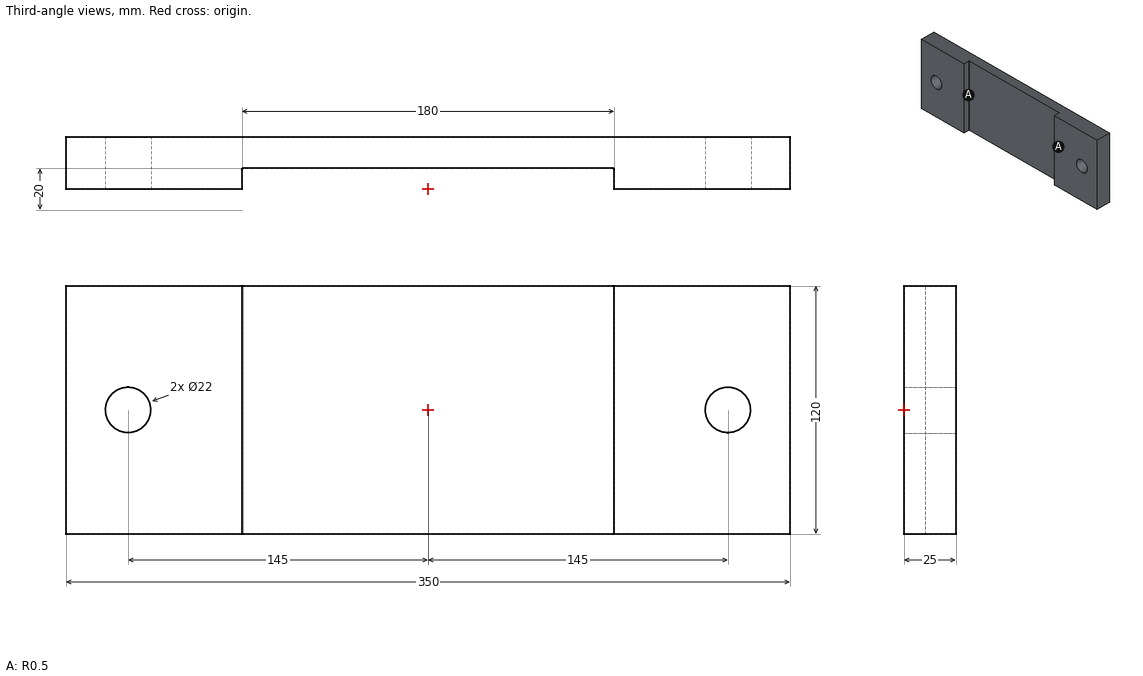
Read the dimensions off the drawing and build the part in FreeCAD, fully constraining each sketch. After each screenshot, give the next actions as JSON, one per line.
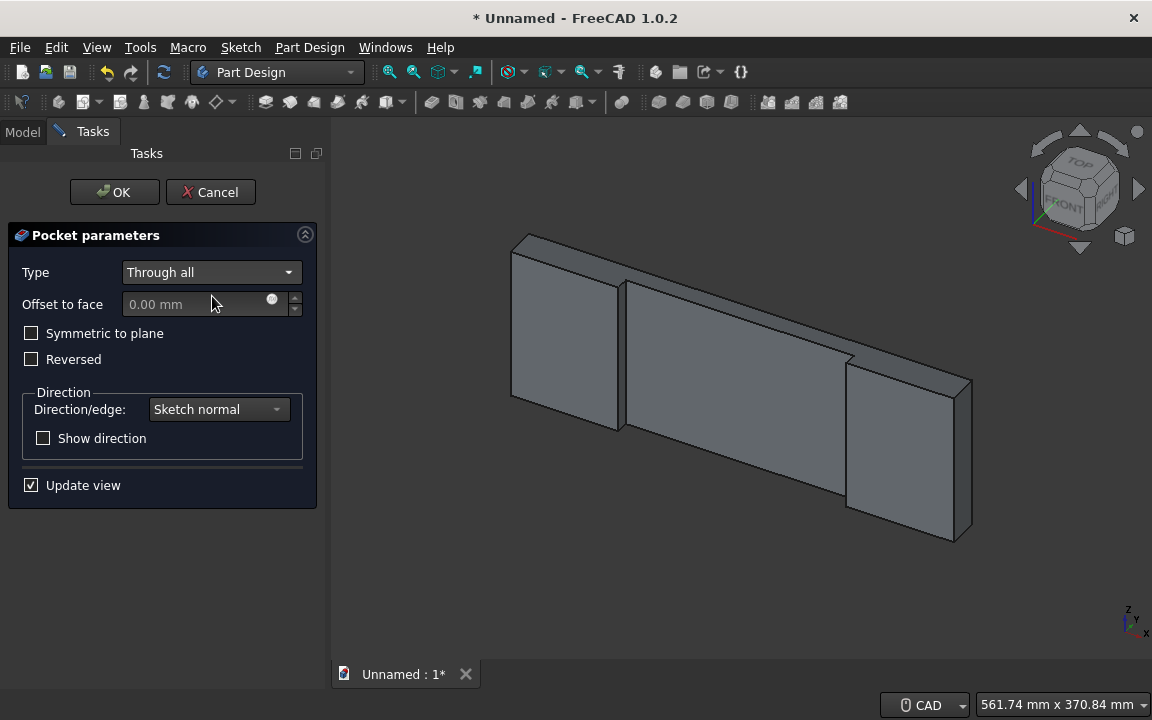
{"action": "left_click", "coordinate": [115, 192]}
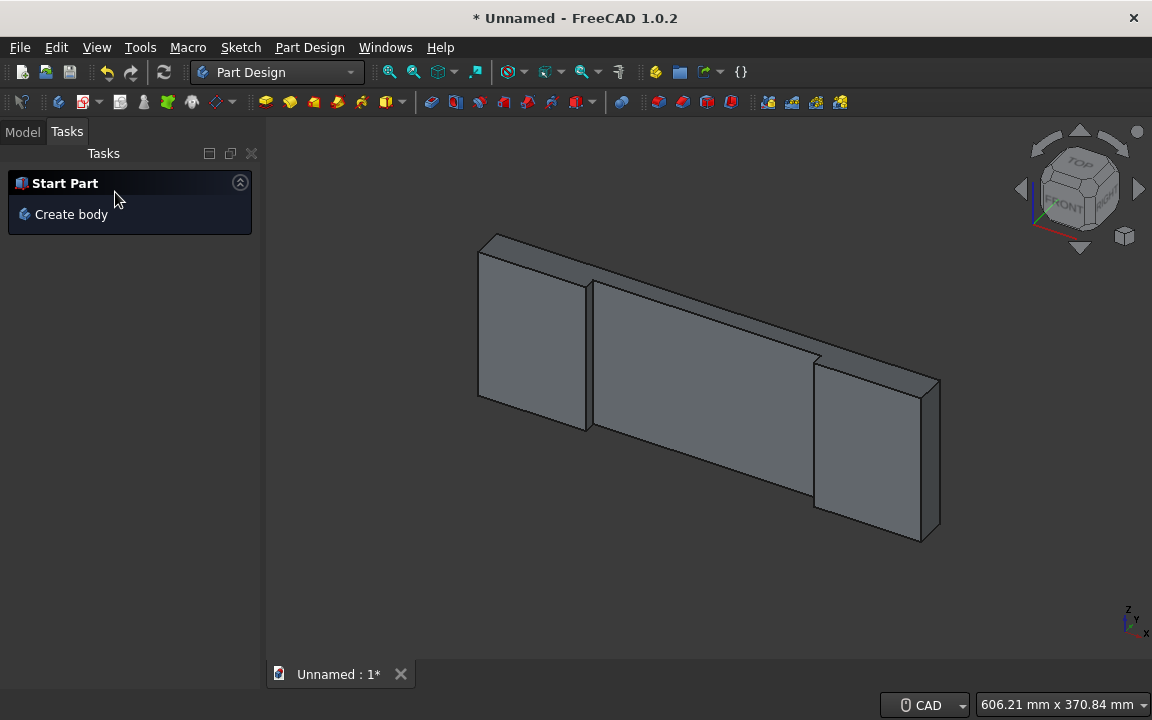
{"action": "key", "text": "4"}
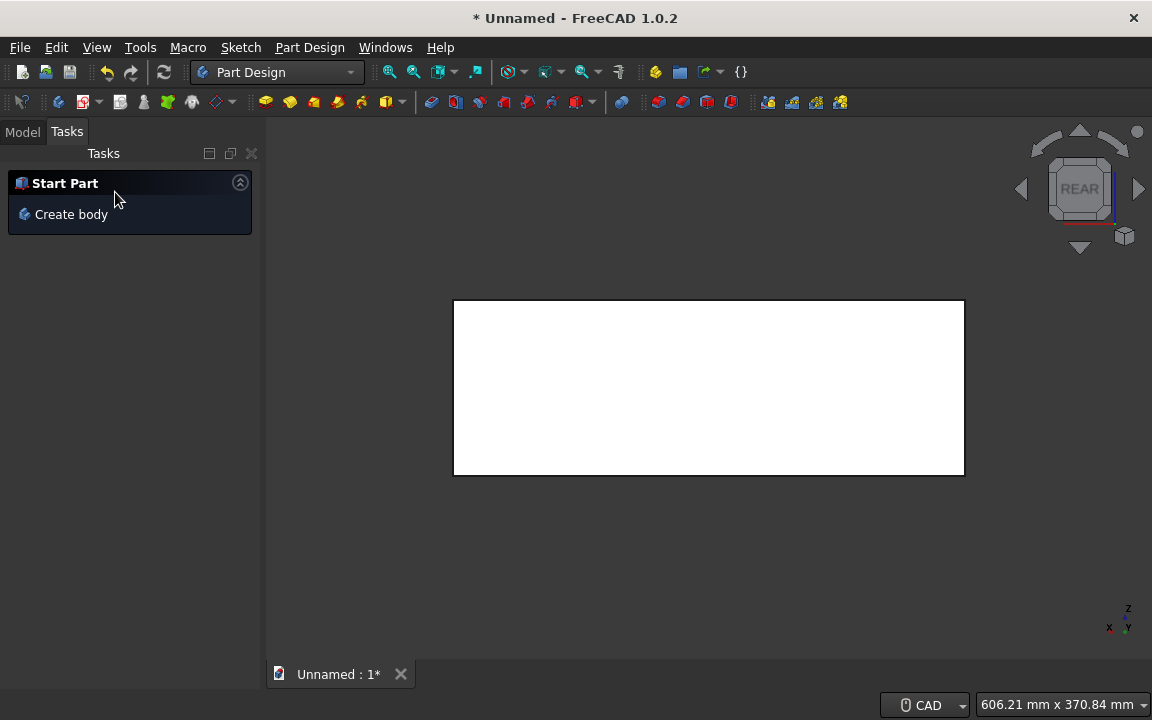
{"action": "left_click", "coordinate": [563, 387]}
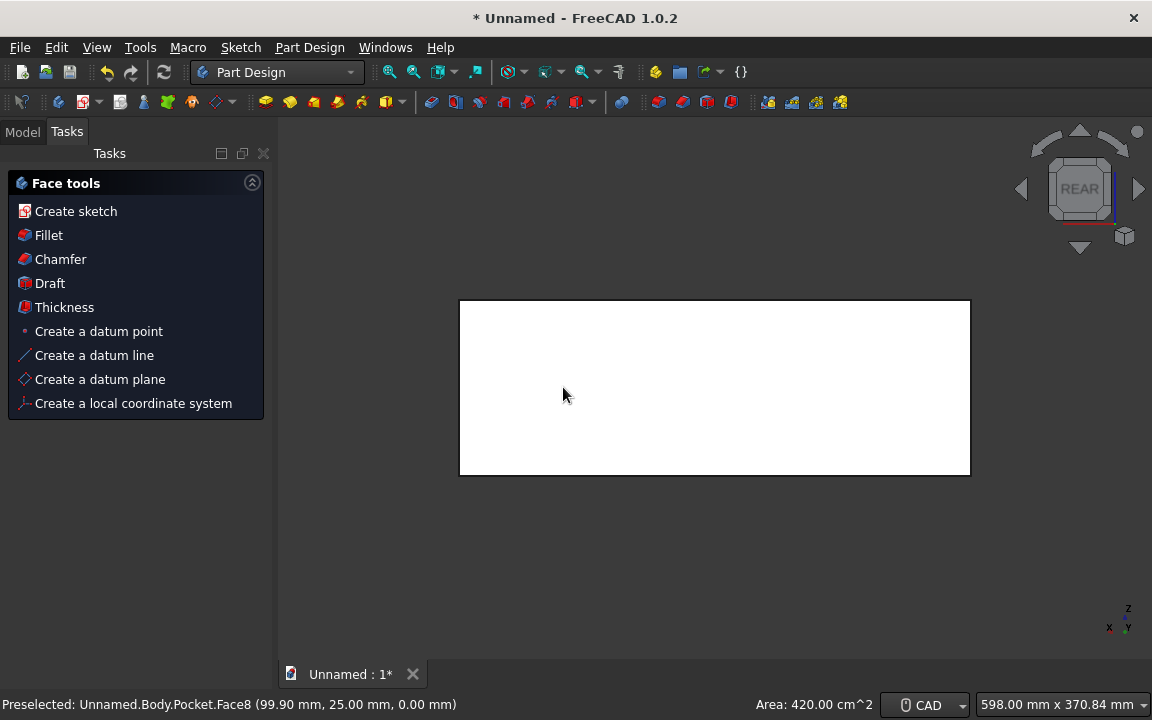
{"action": "left_click", "coordinate": [84, 102]}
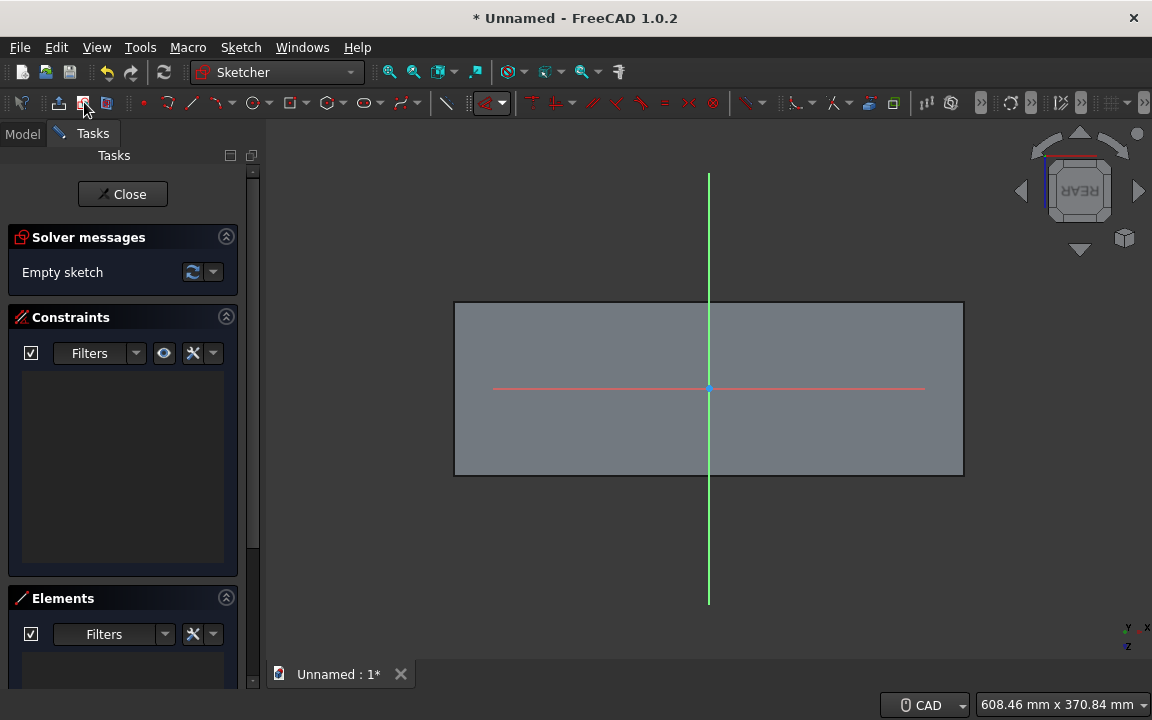
{"action": "left_click", "coordinate": [254, 104]}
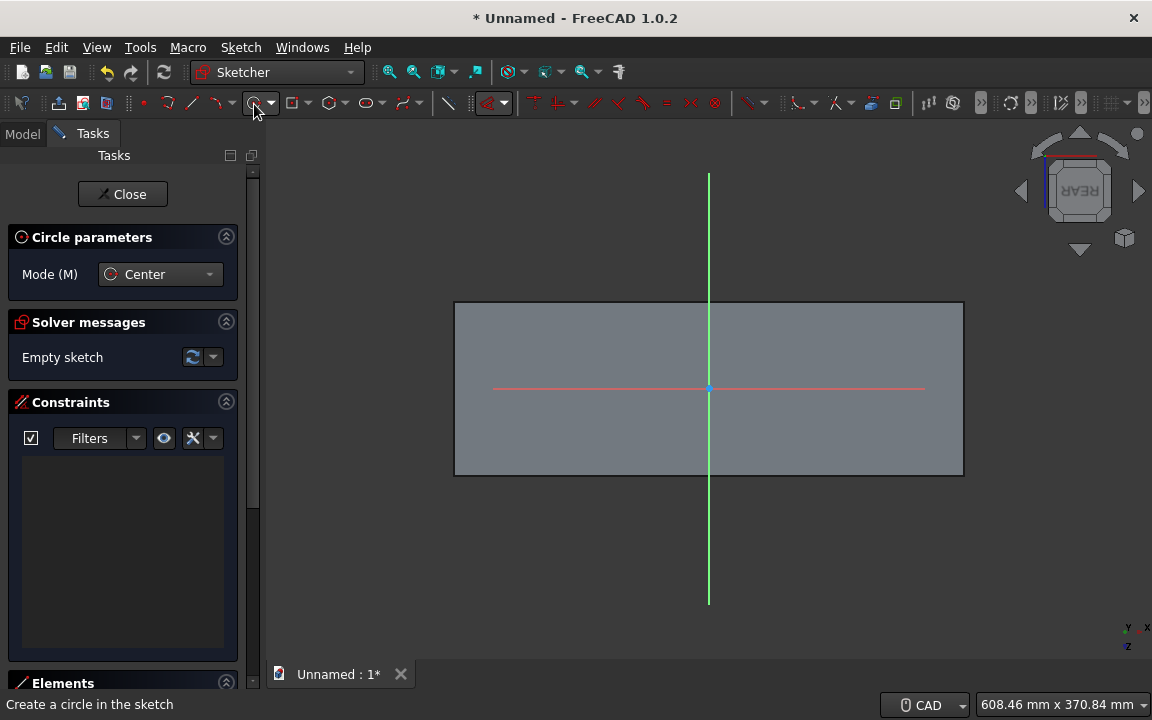
{"action": "scroll", "coordinate": [498, 389], "scroll_direction": "up", "scroll_amount": 2}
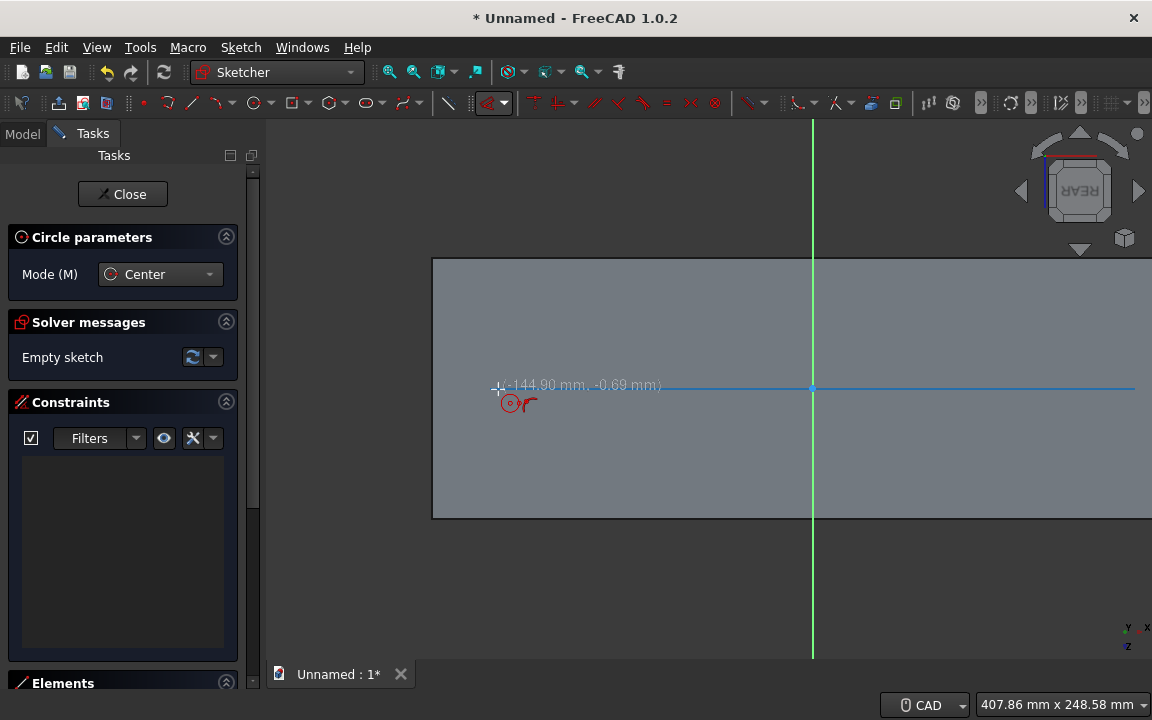
{"action": "left_click", "coordinate": [498, 389]}
{"action": "mouse_move", "coordinate": [515, 372]}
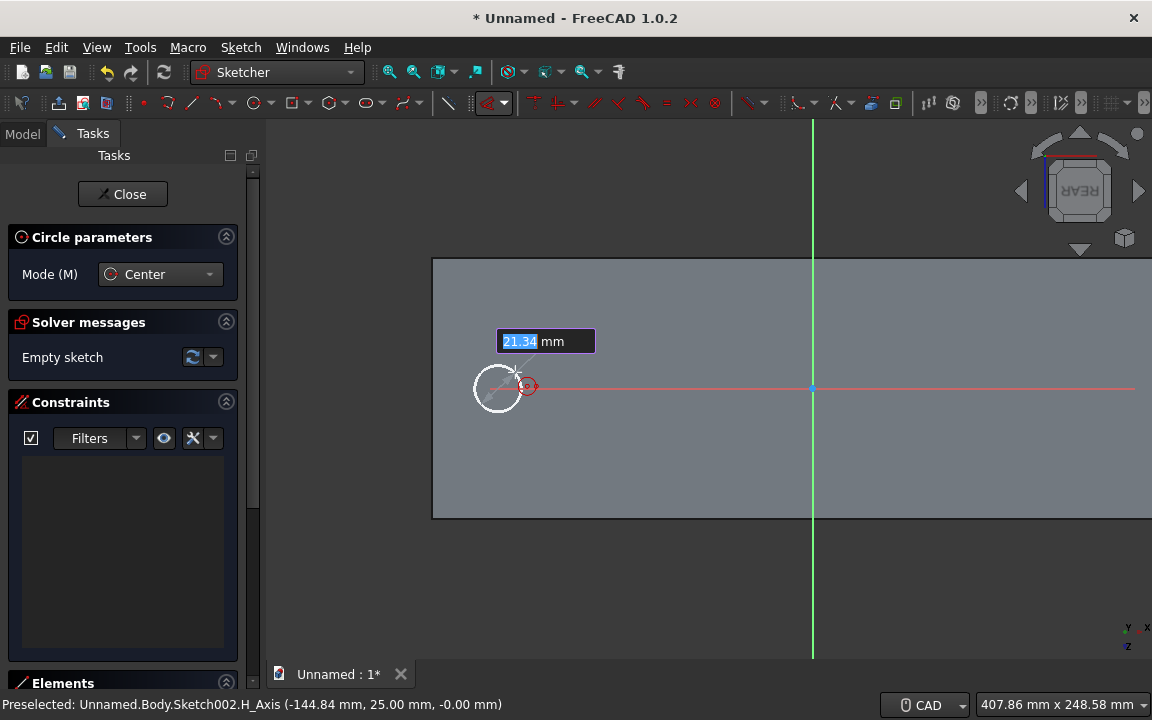
{"action": "type", "text": "22"}
{"action": "key", "text": "Return"}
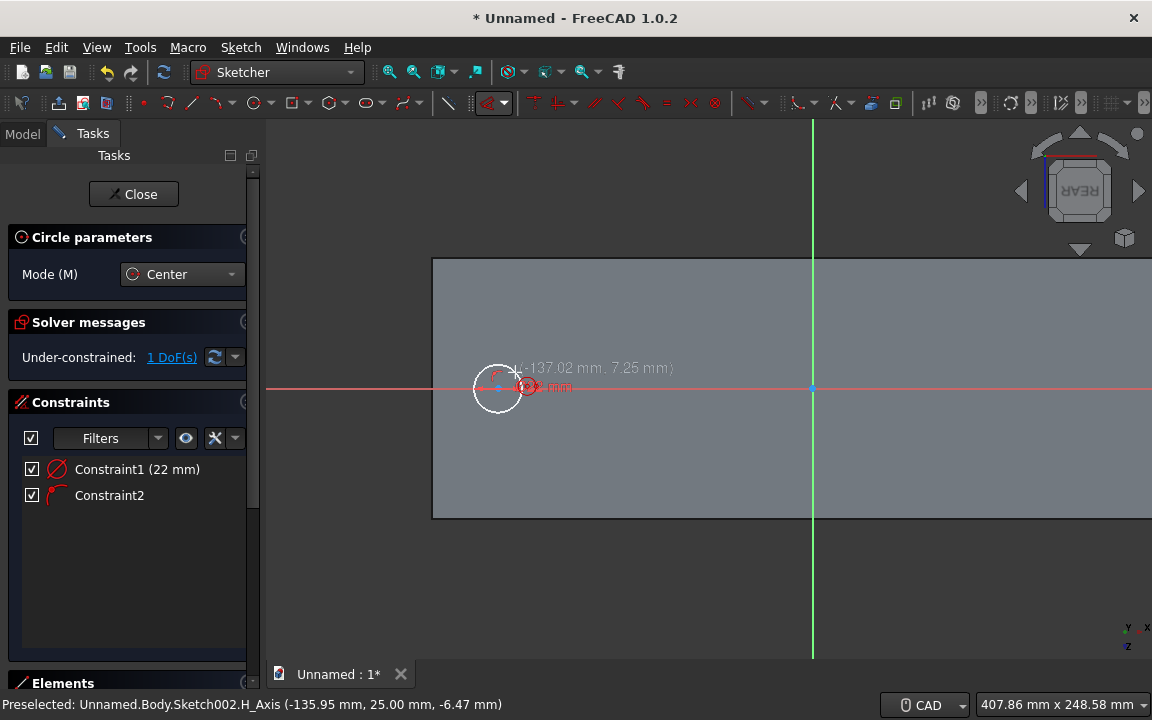
{"action": "scroll", "coordinate": [294, 390], "scroll_direction": "down", "scroll_amount": 2}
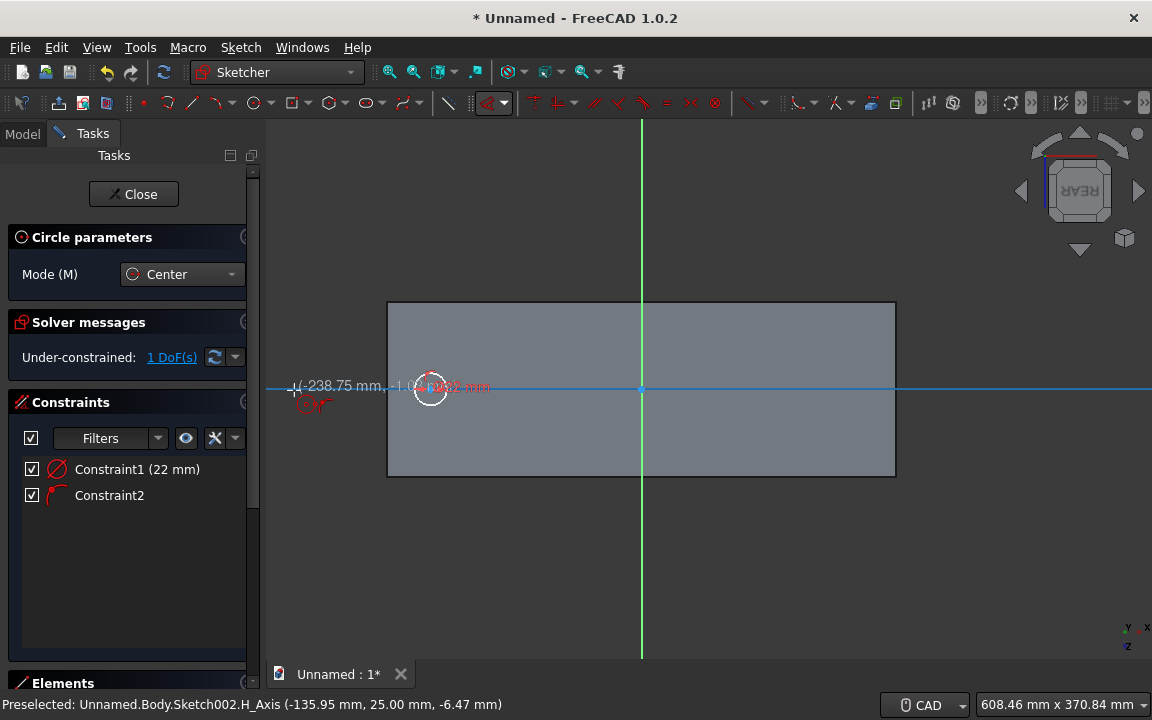
{"action": "scroll", "coordinate": [853, 389], "scroll_direction": "up", "scroll_amount": 2}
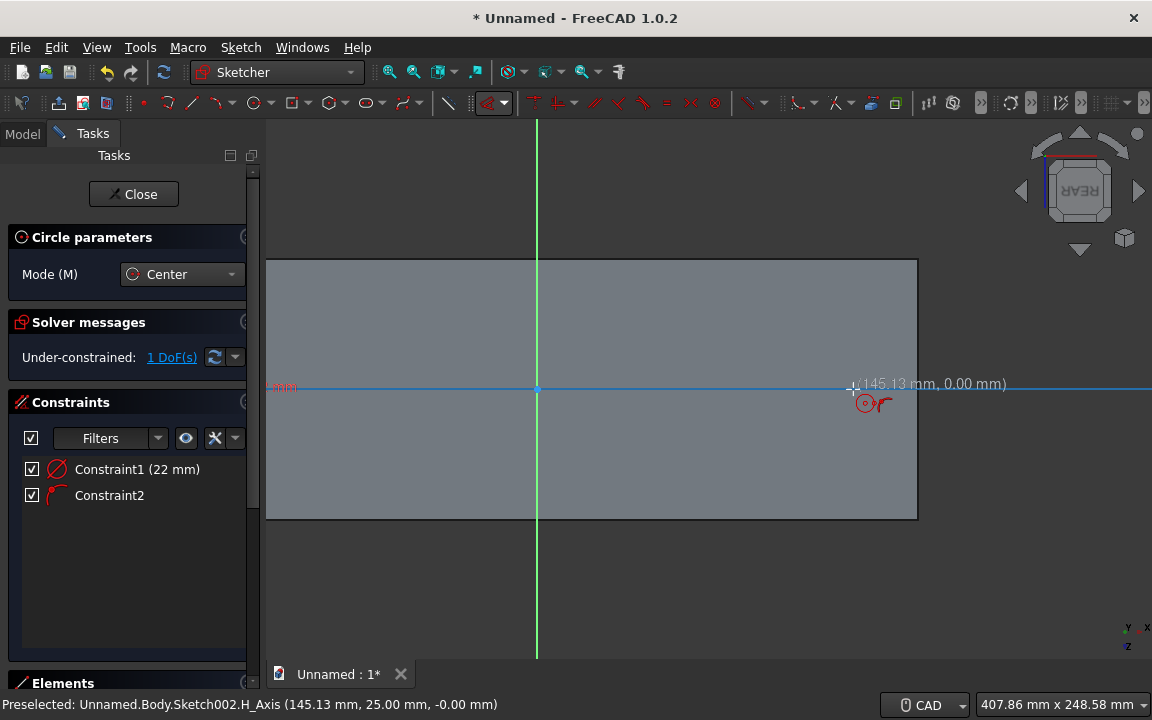
{"action": "left_click", "coordinate": [852, 389]}
{"action": "mouse_move", "coordinate": [869, 372]}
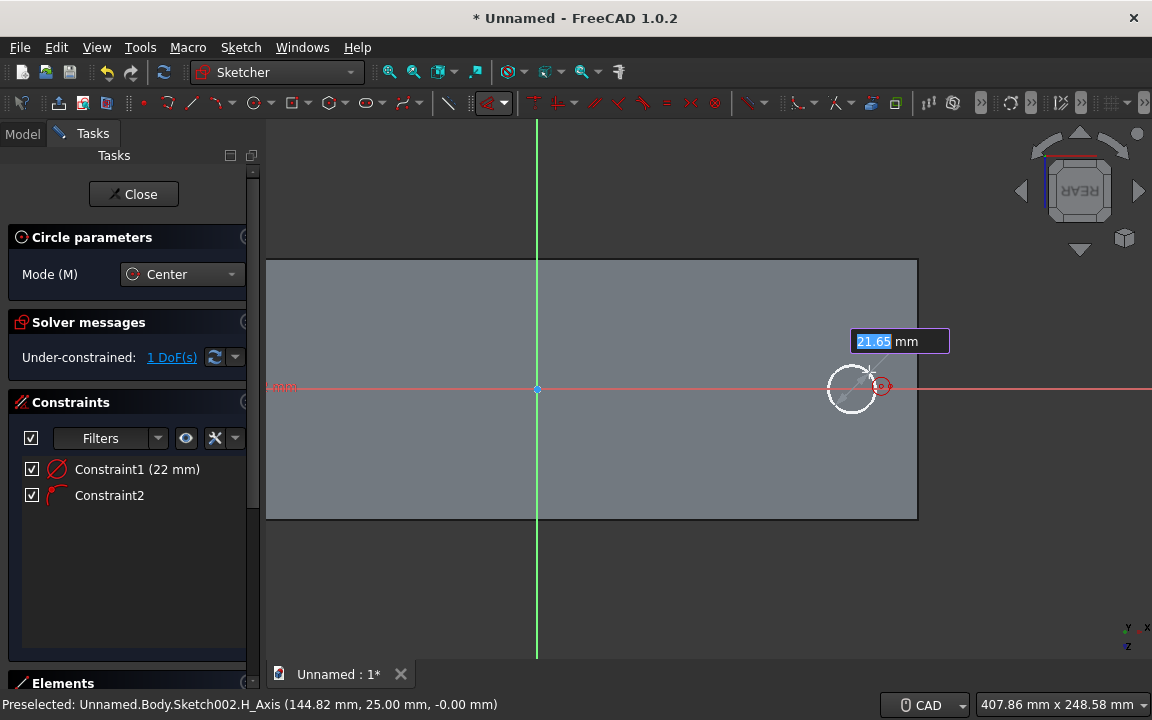
{"action": "type", "text": "22"}
{"action": "key", "text": "Return"}
{"action": "key", "text": "Escape"}